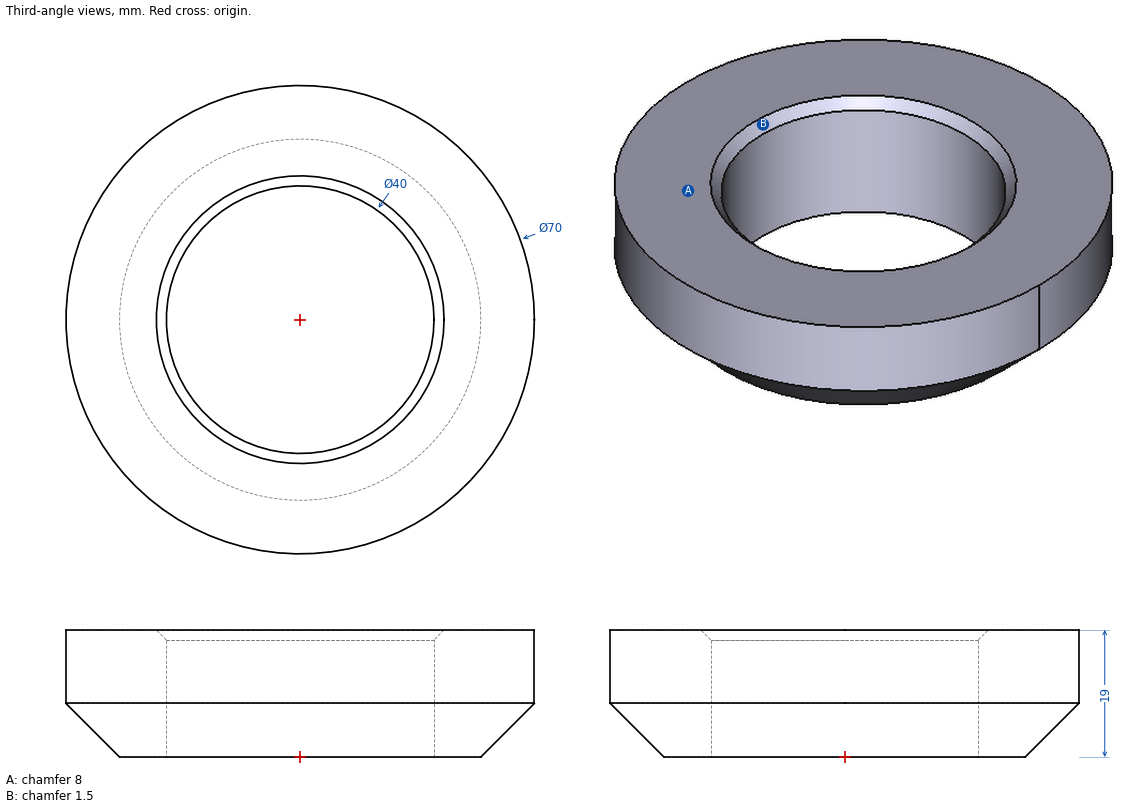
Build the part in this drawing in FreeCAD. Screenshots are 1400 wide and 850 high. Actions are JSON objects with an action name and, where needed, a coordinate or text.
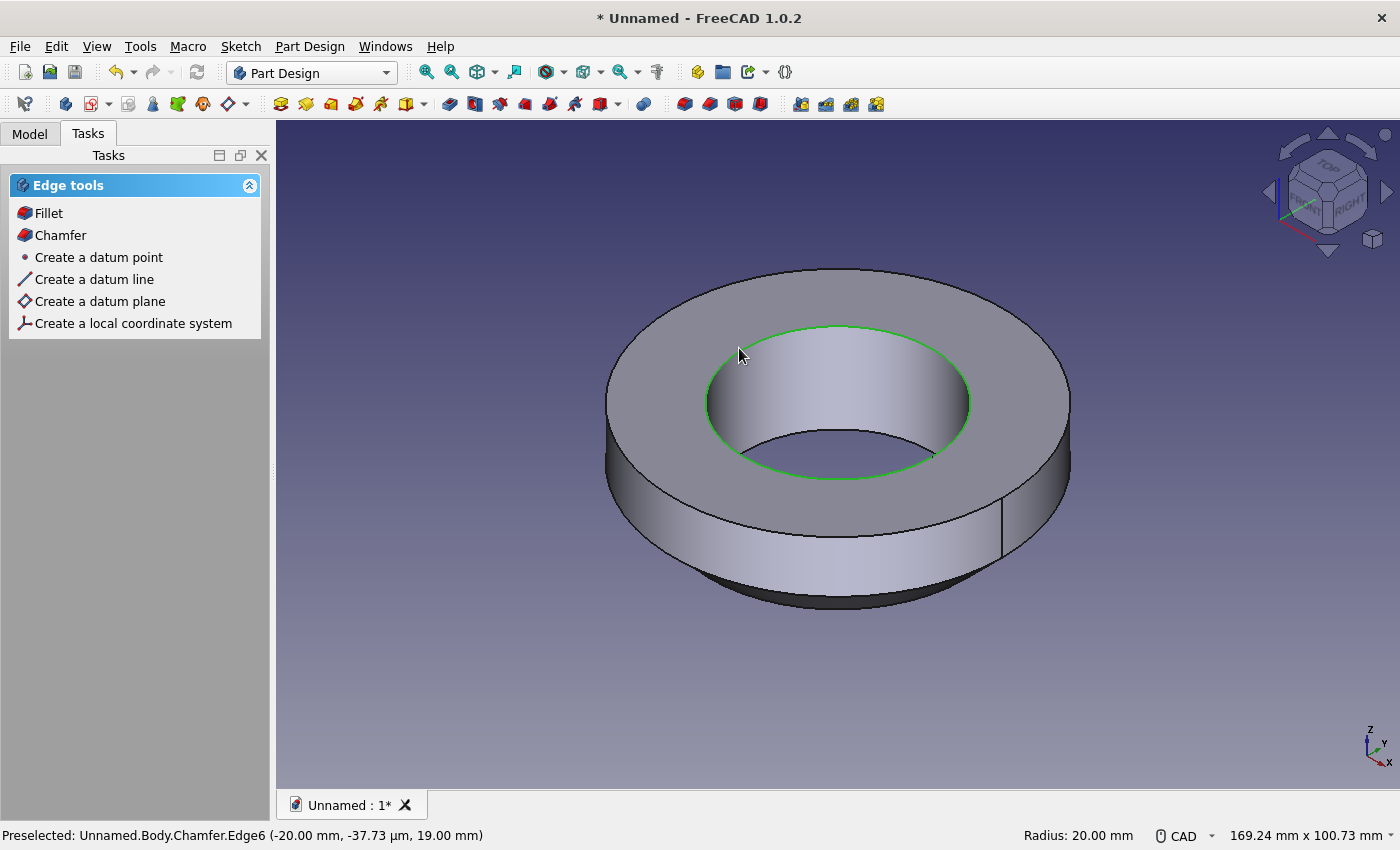
{"action": "left_click", "coordinate": [710, 104]}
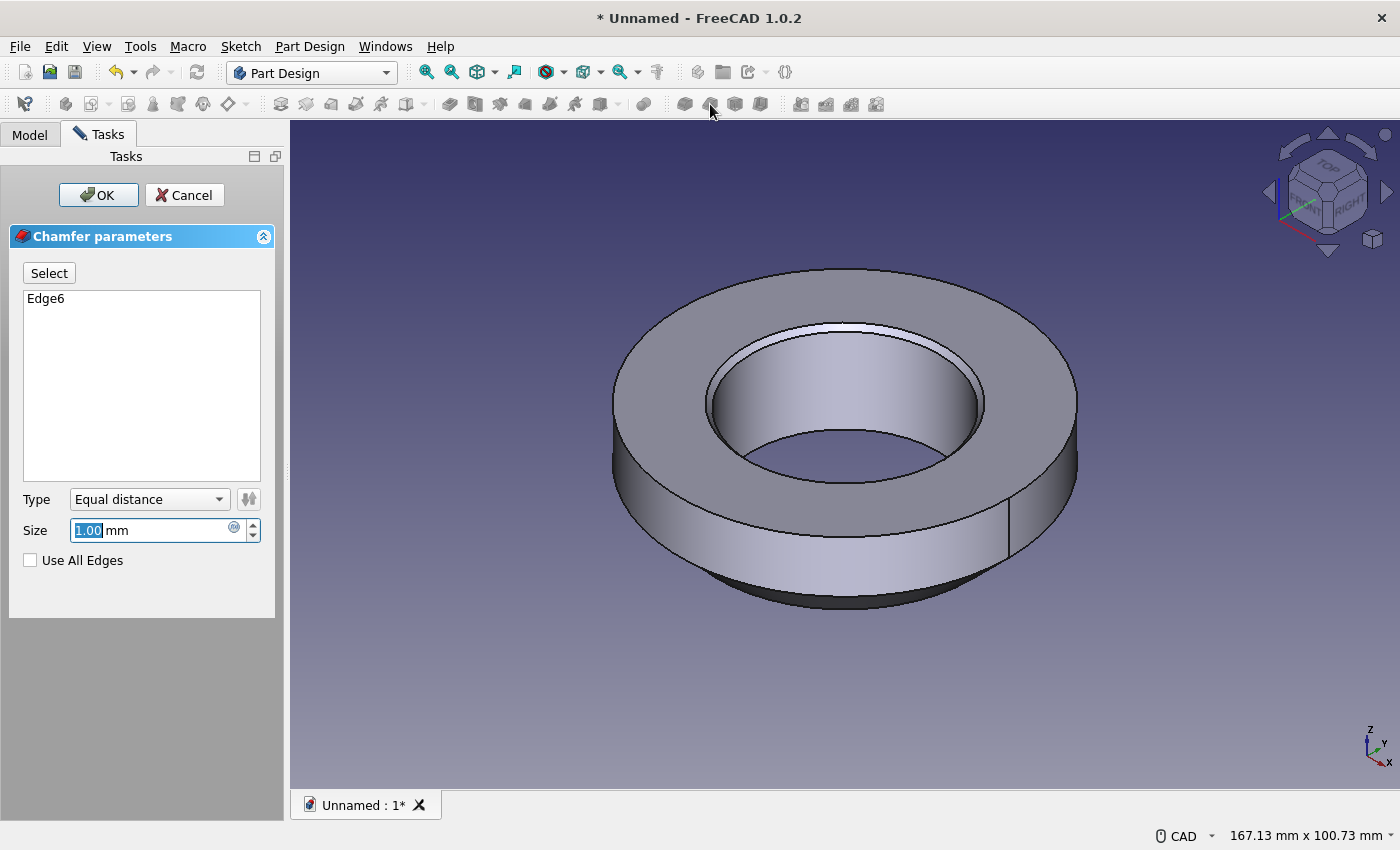
{"action": "type", "text": "1.5"}
{"action": "key", "text": "Tab"}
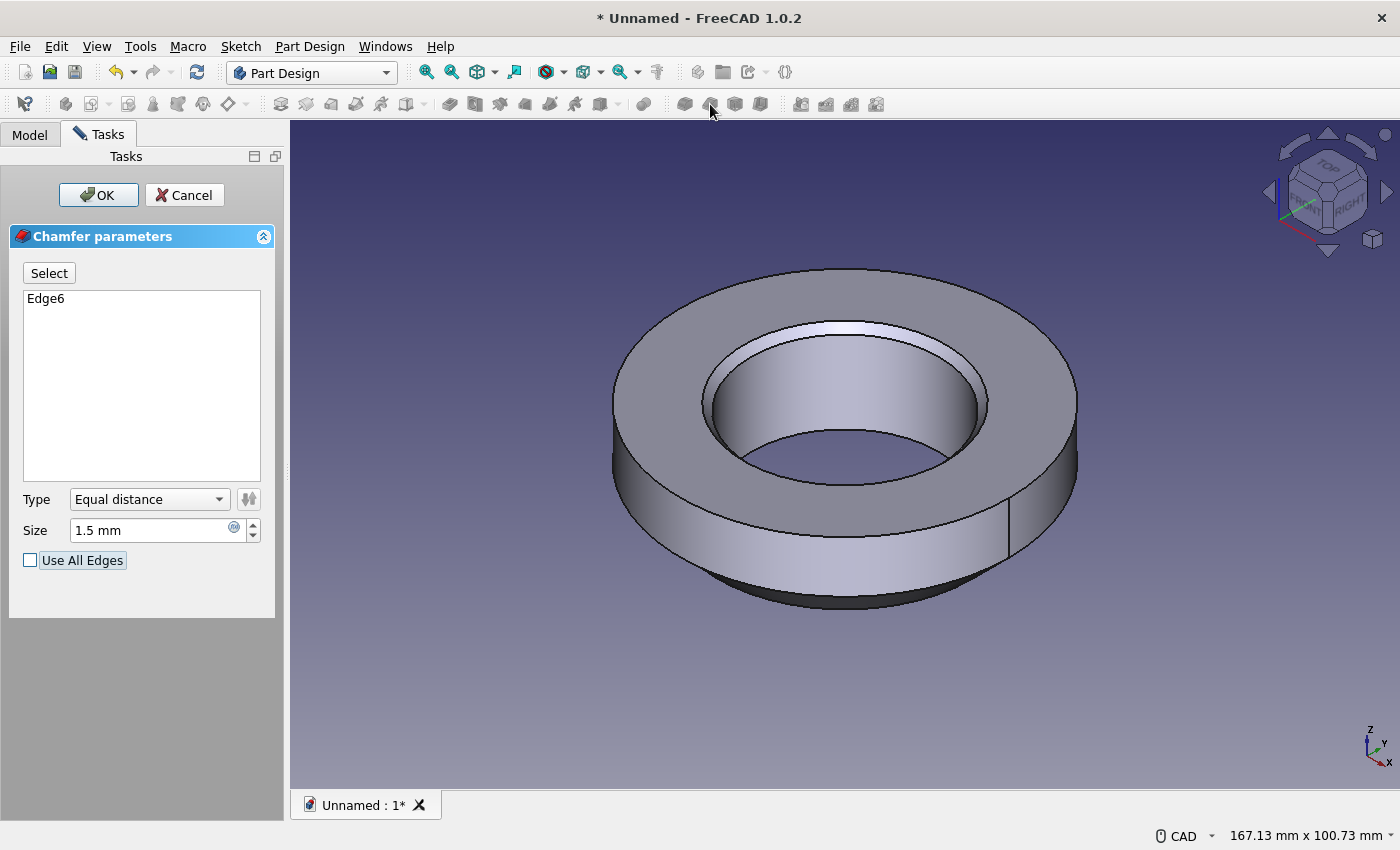
{"action": "left_click", "coordinate": [99, 195]}